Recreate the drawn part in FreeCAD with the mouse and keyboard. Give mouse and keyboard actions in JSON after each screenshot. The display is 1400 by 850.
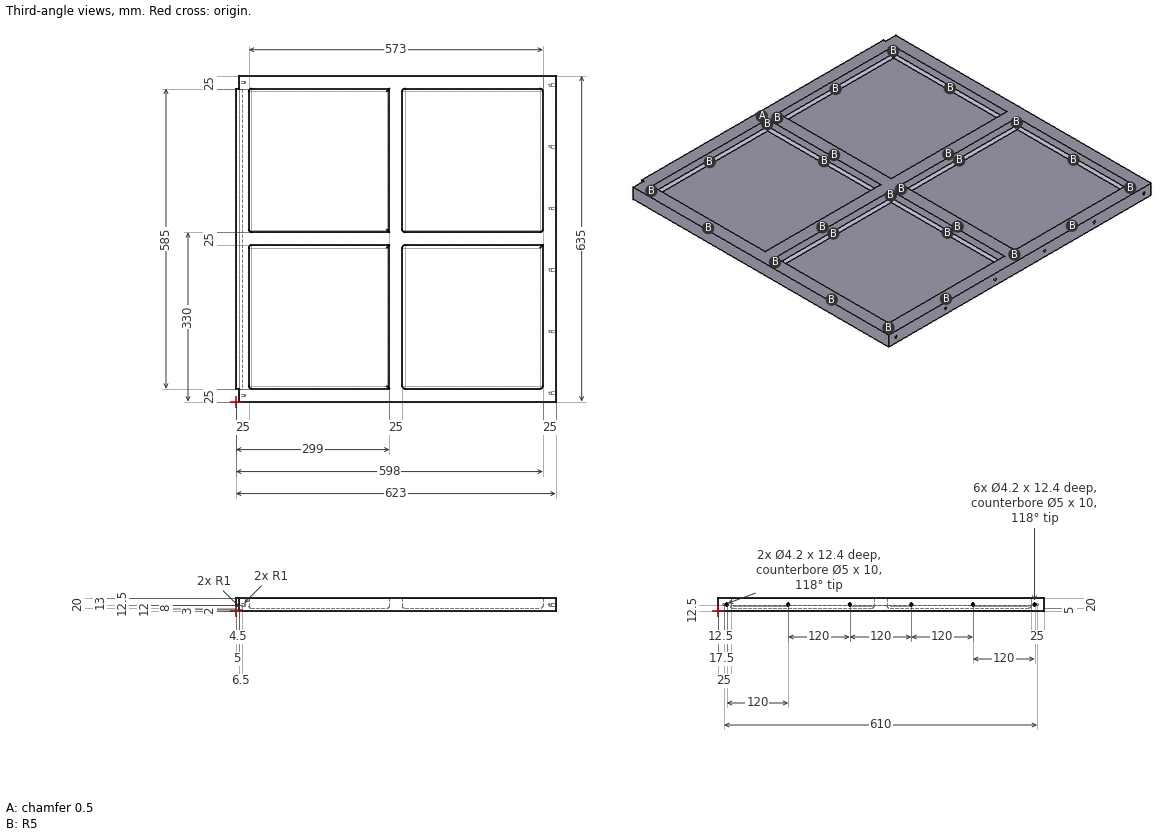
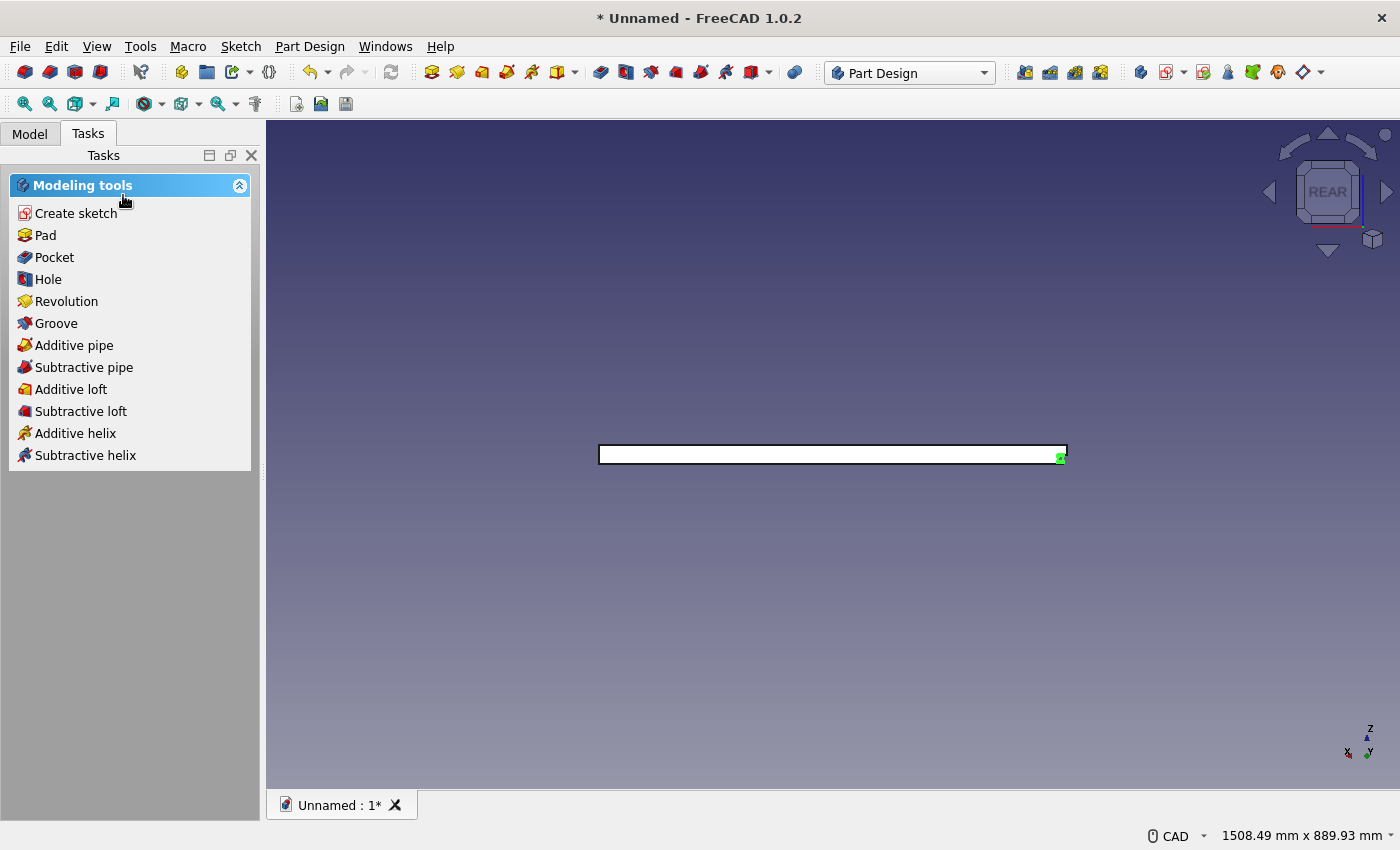
{"action": "left_click", "coordinate": [432, 72]}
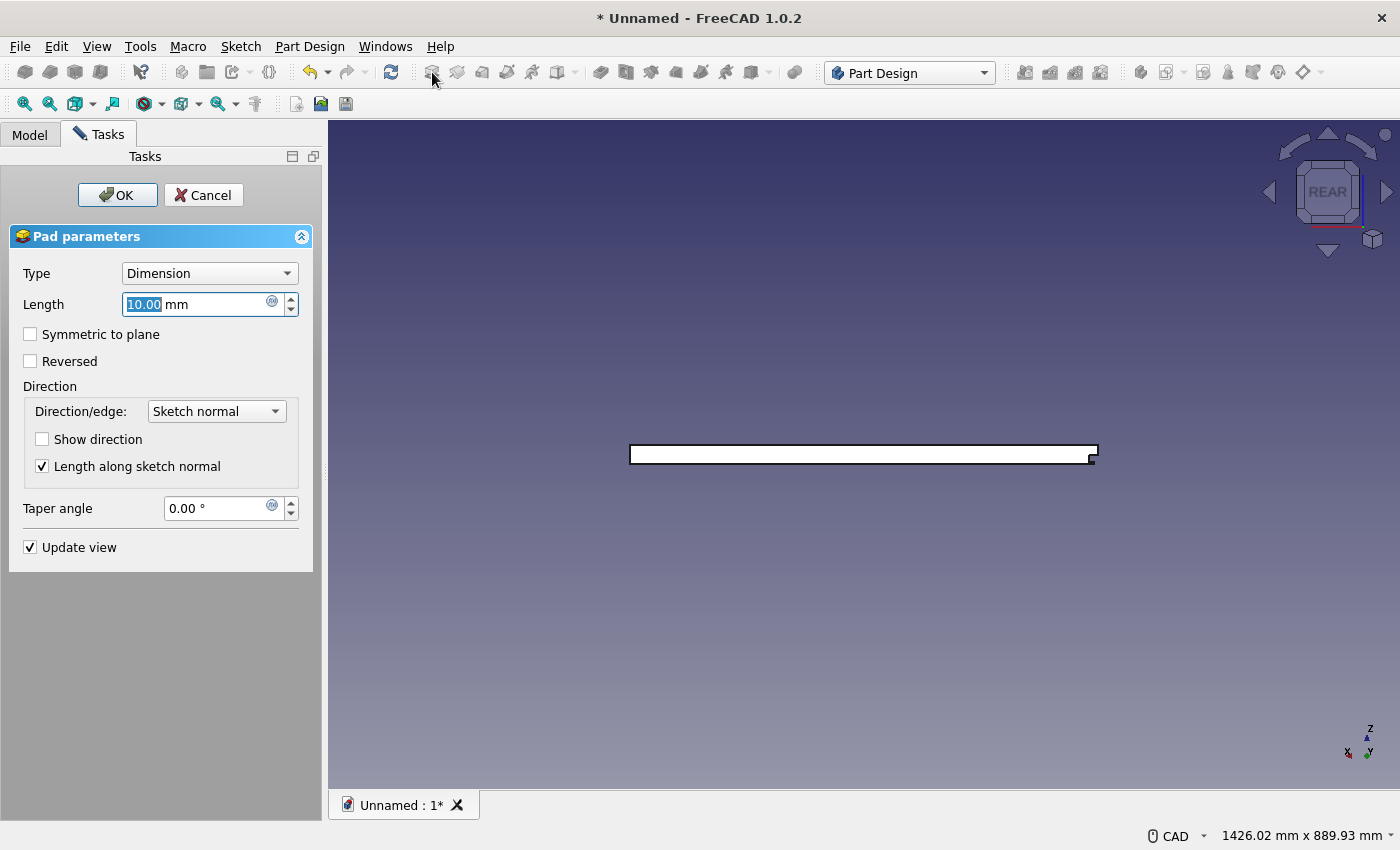
{"action": "type", "text": "25"}
{"action": "key", "text": "Tab"}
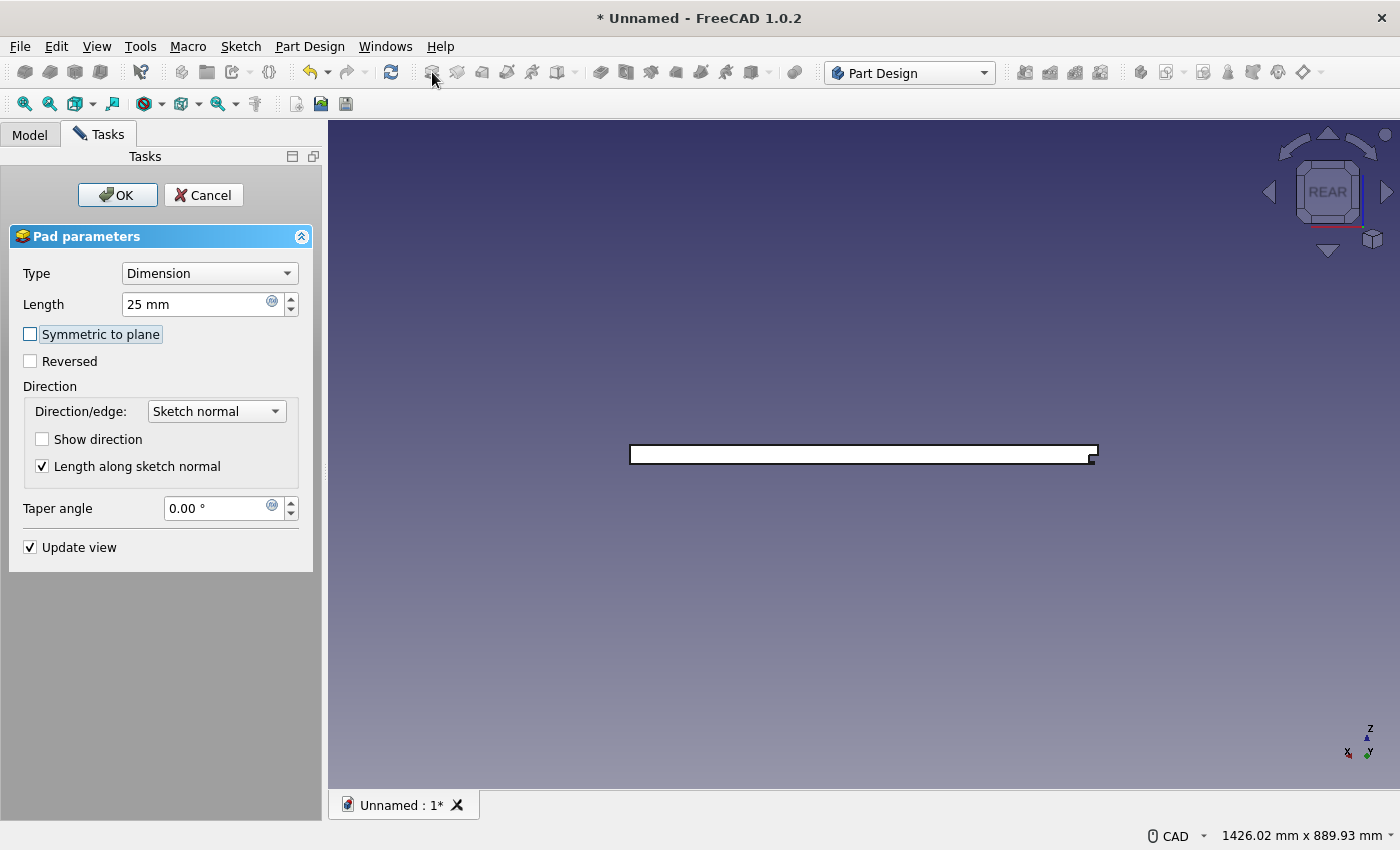
{"action": "left_click", "coordinate": [31, 361]}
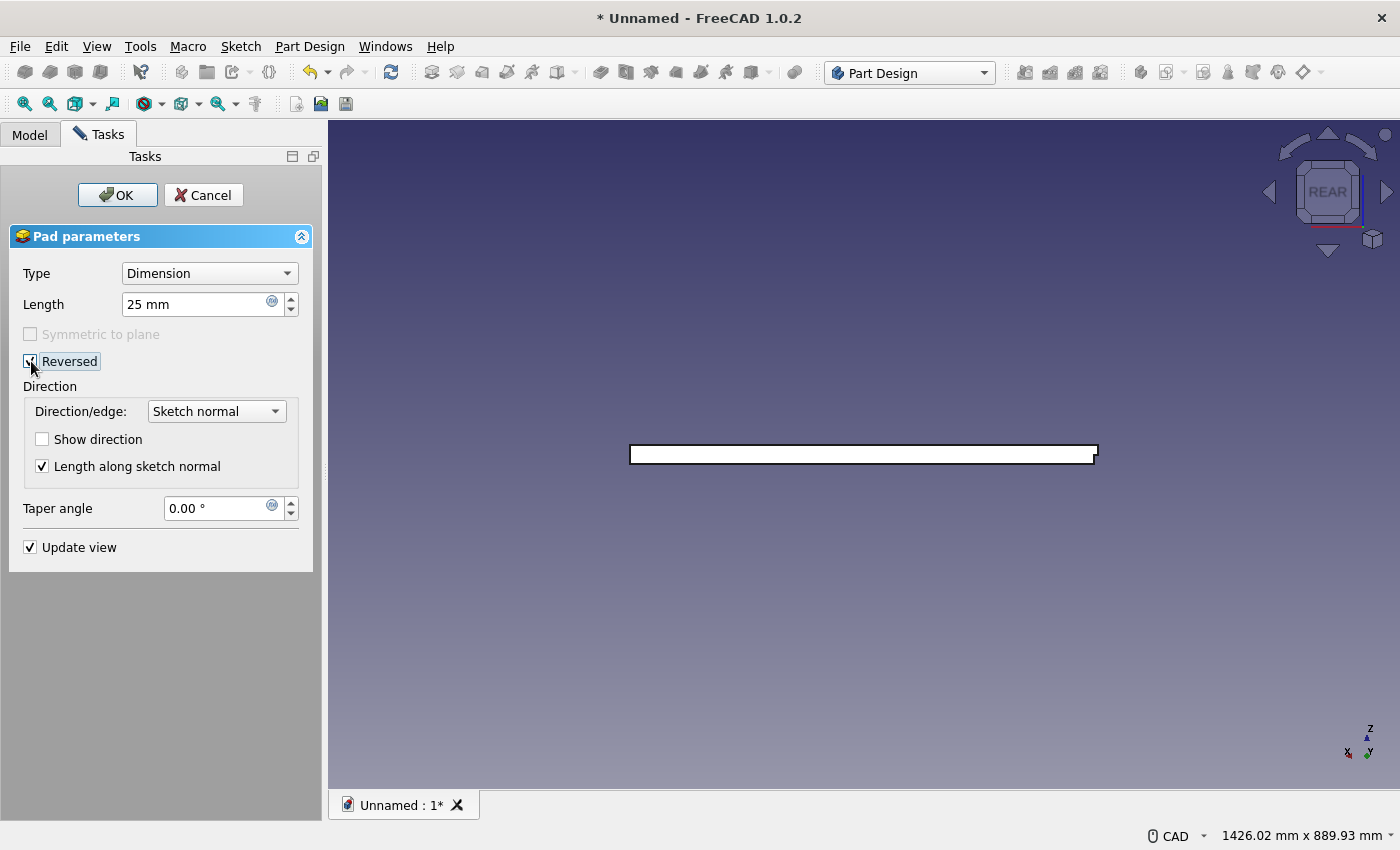
{"action": "left_click", "coordinate": [118, 195]}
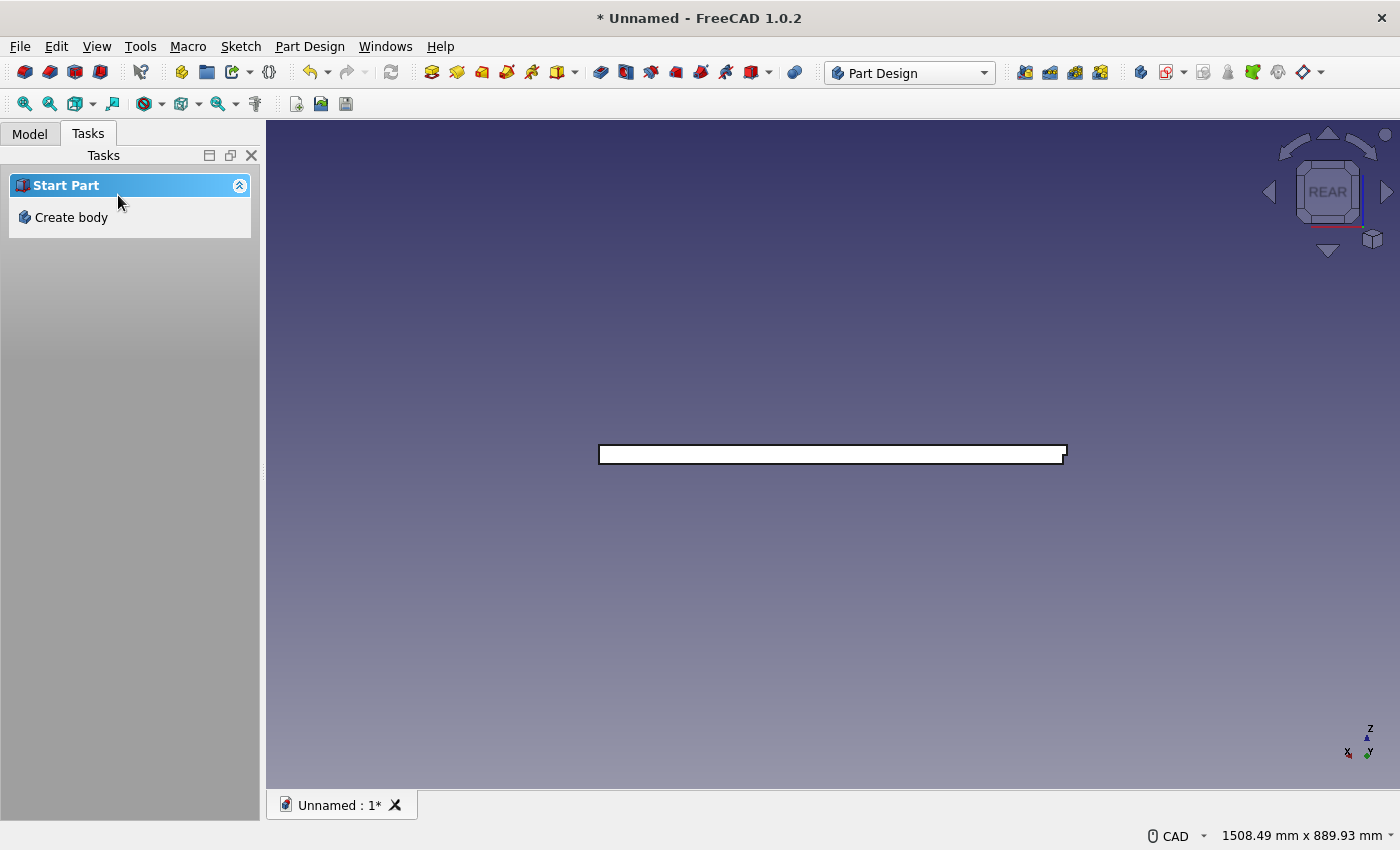
{"action": "left_click", "coordinate": [25, 104]}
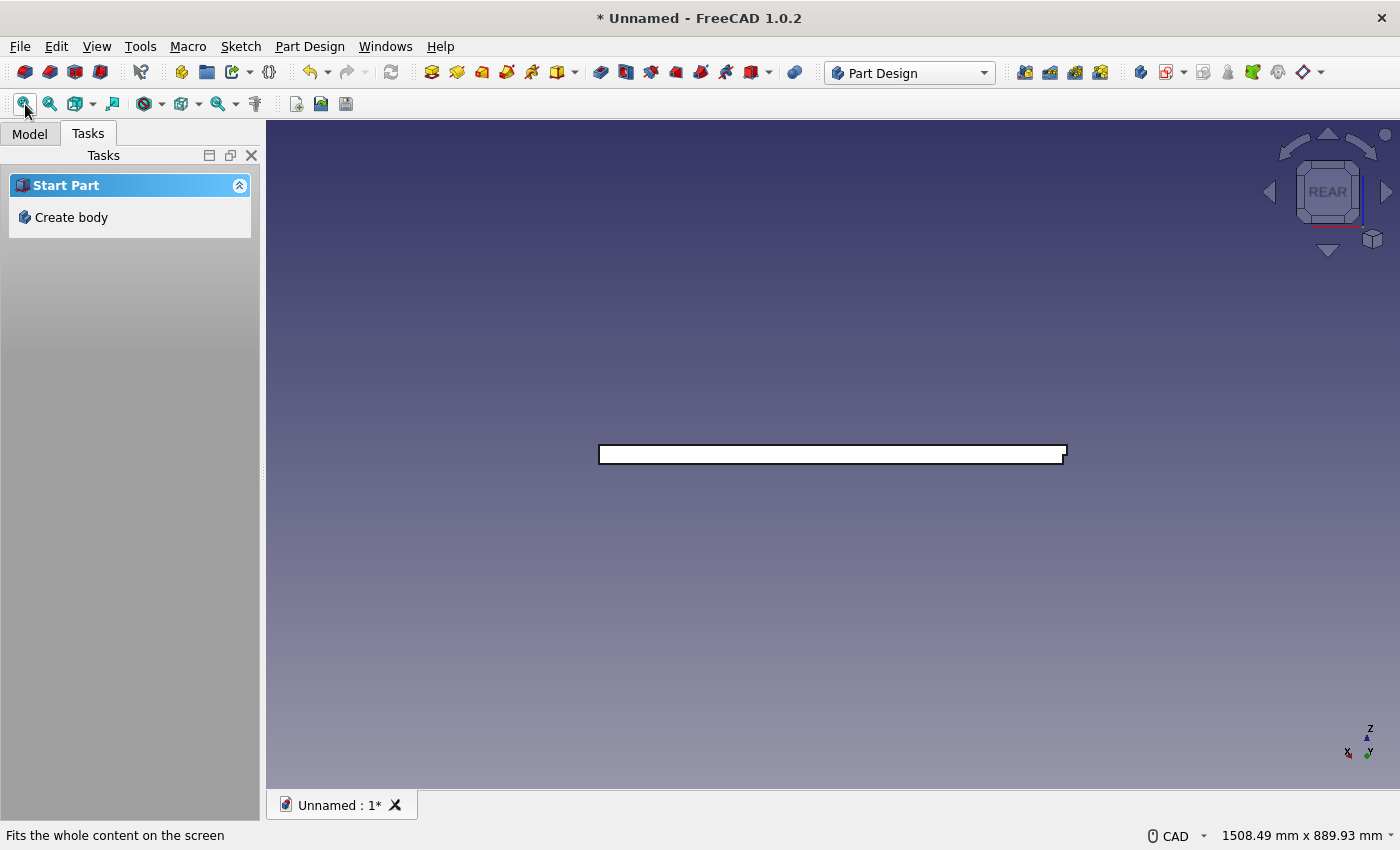
{"action": "left_click", "coordinate": [632, 453]}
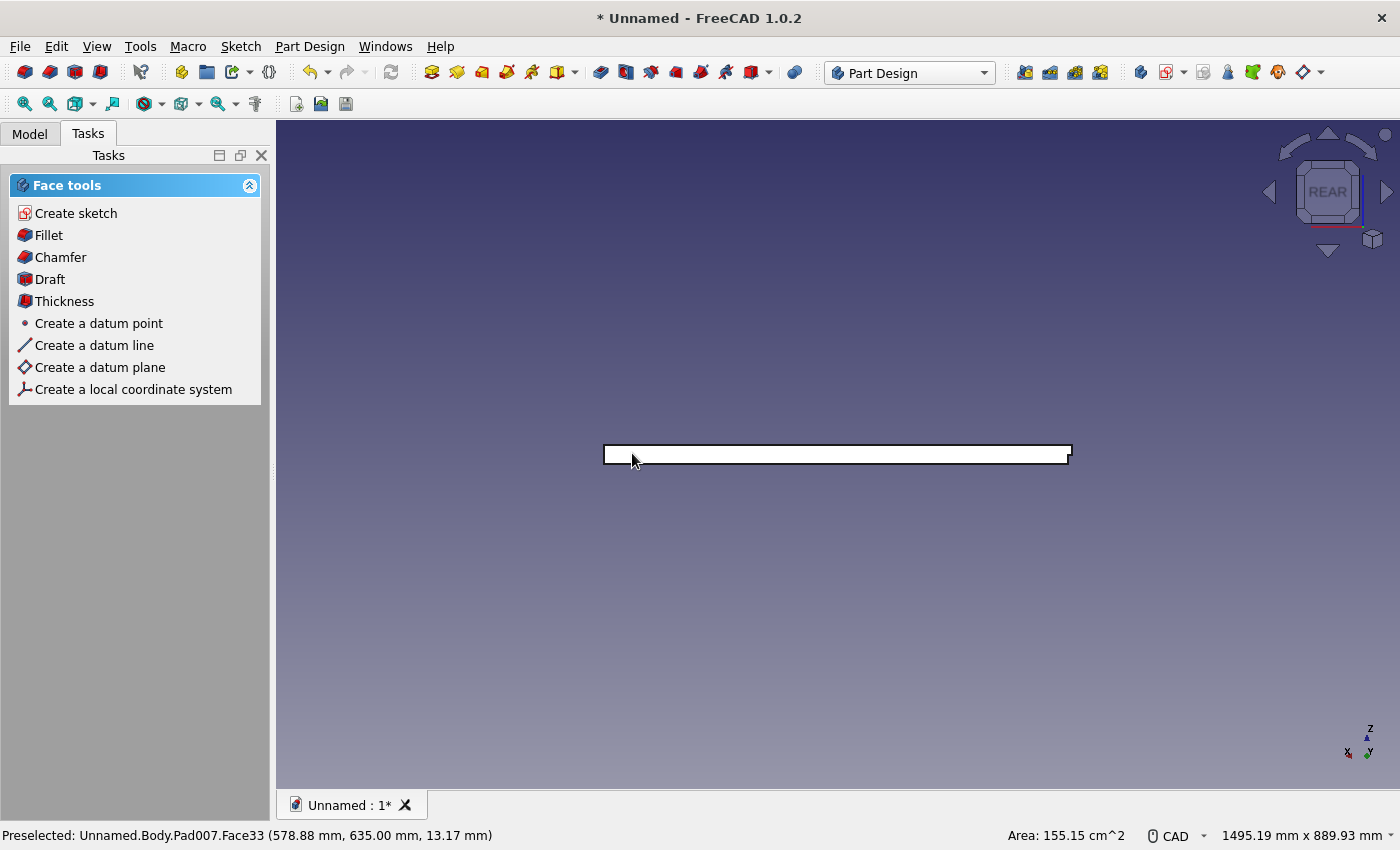
{"action": "left_click", "coordinate": [1166, 72]}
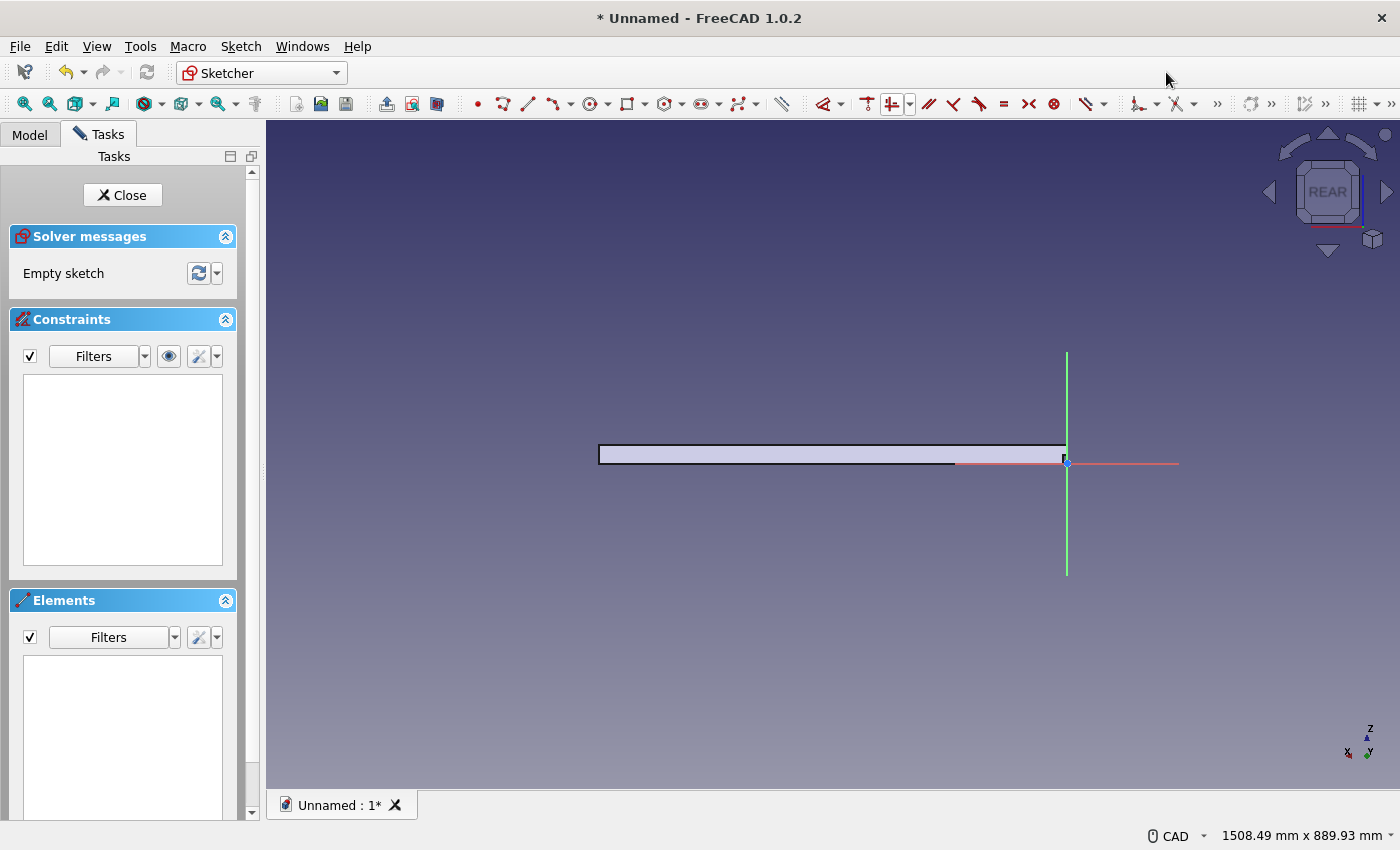
{"action": "scroll", "coordinate": [1081, 455], "scroll_direction": "up", "scroll_amount": 15}